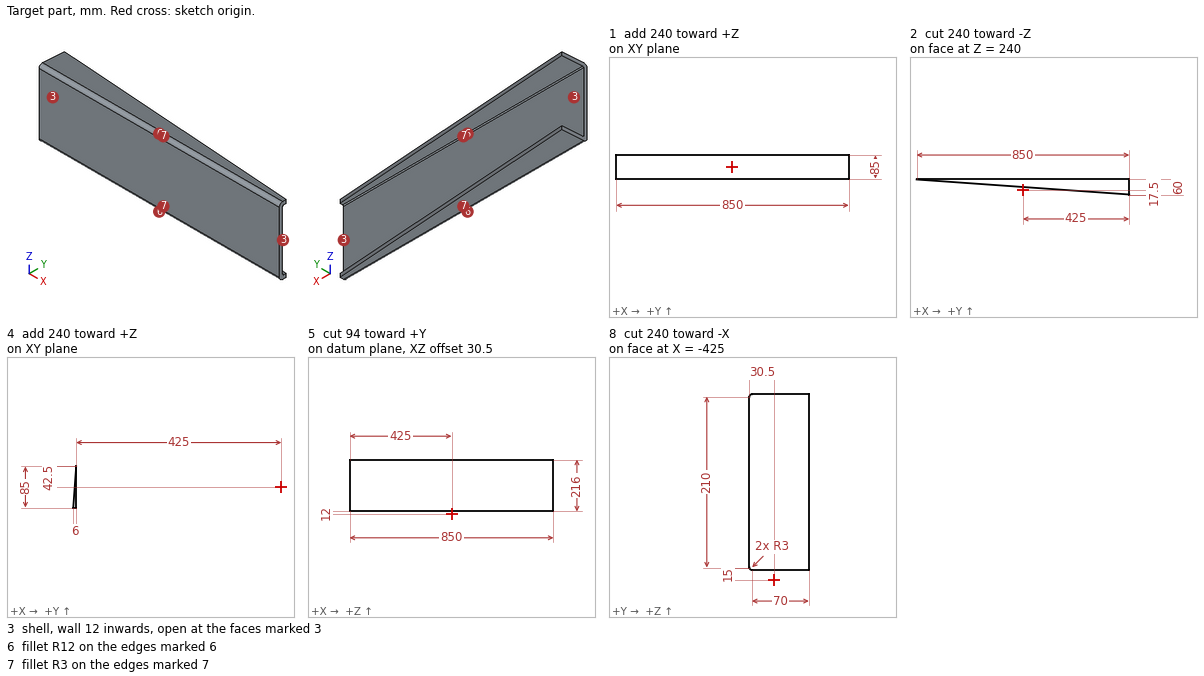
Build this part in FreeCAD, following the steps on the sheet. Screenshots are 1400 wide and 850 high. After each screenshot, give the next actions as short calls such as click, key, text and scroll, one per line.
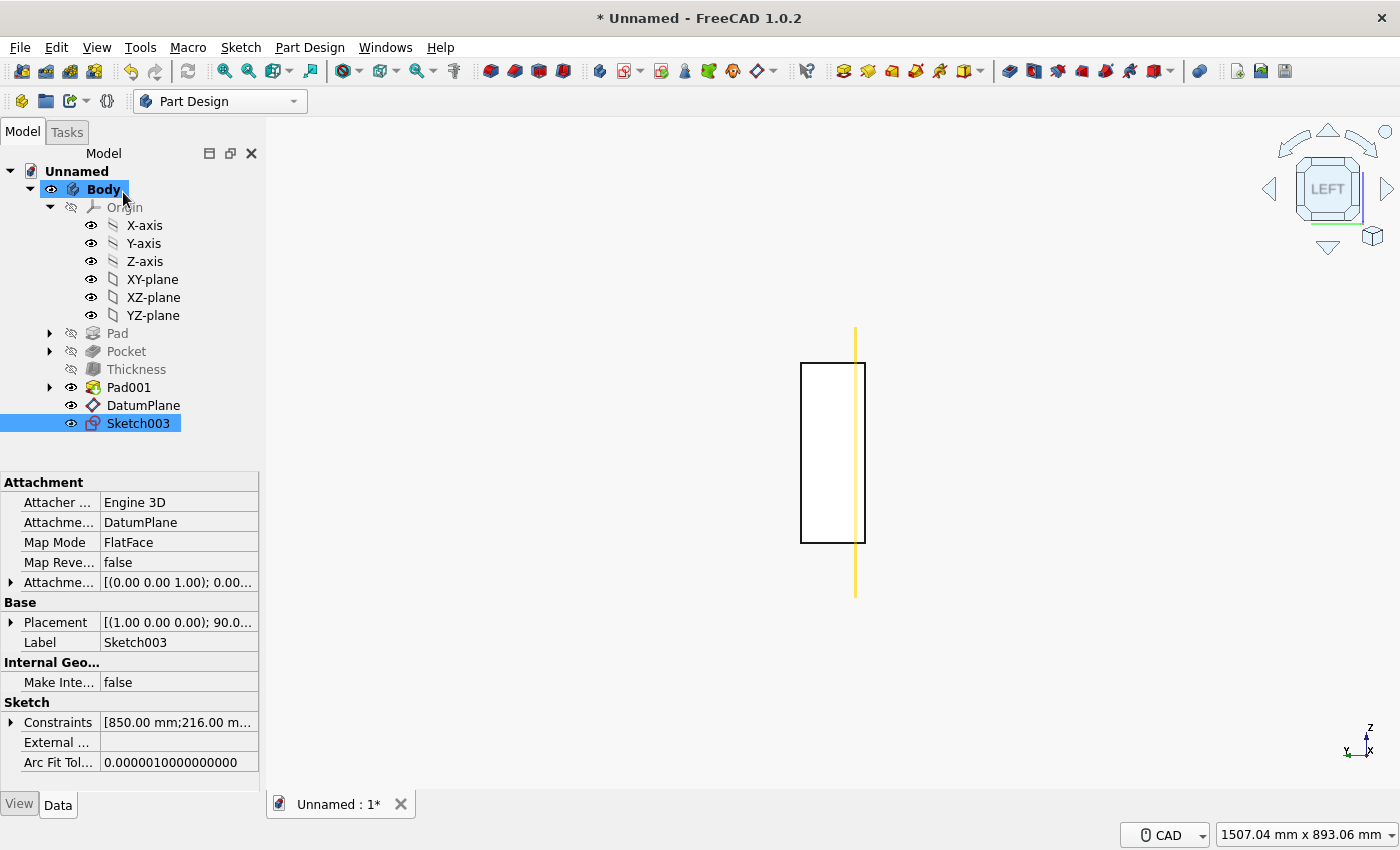
click(1010, 72)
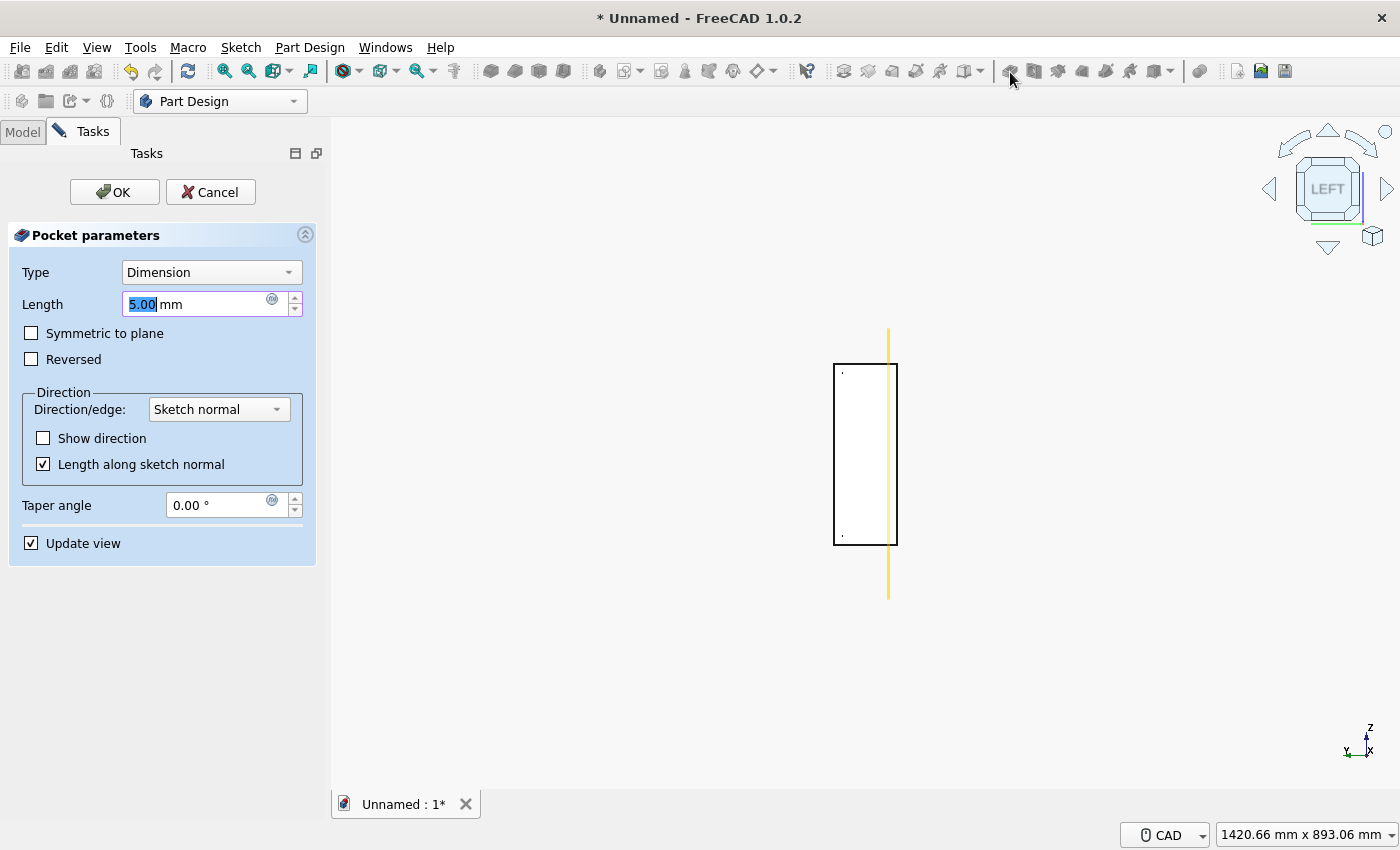
text(94)
key(Tab)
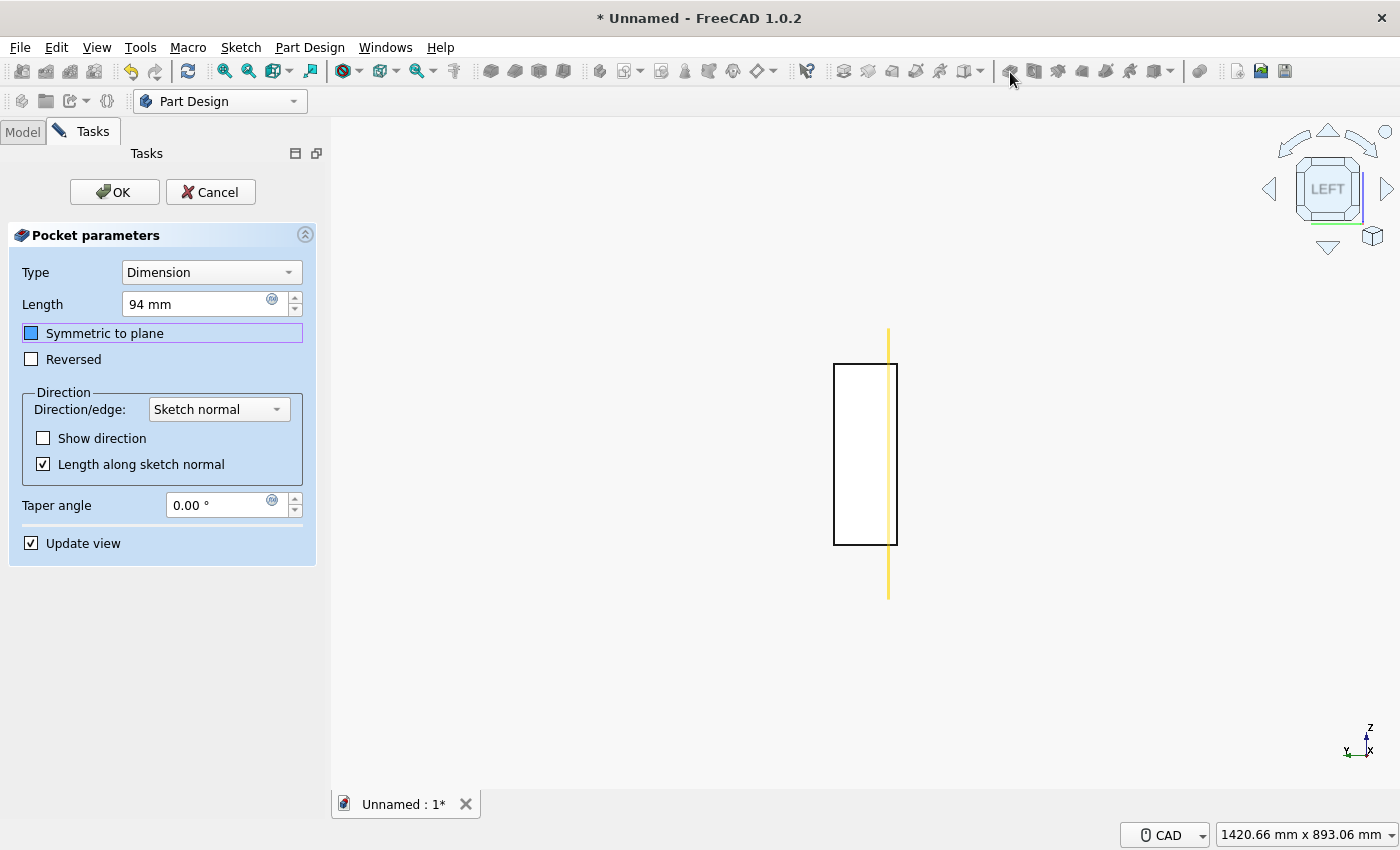
click(115, 192)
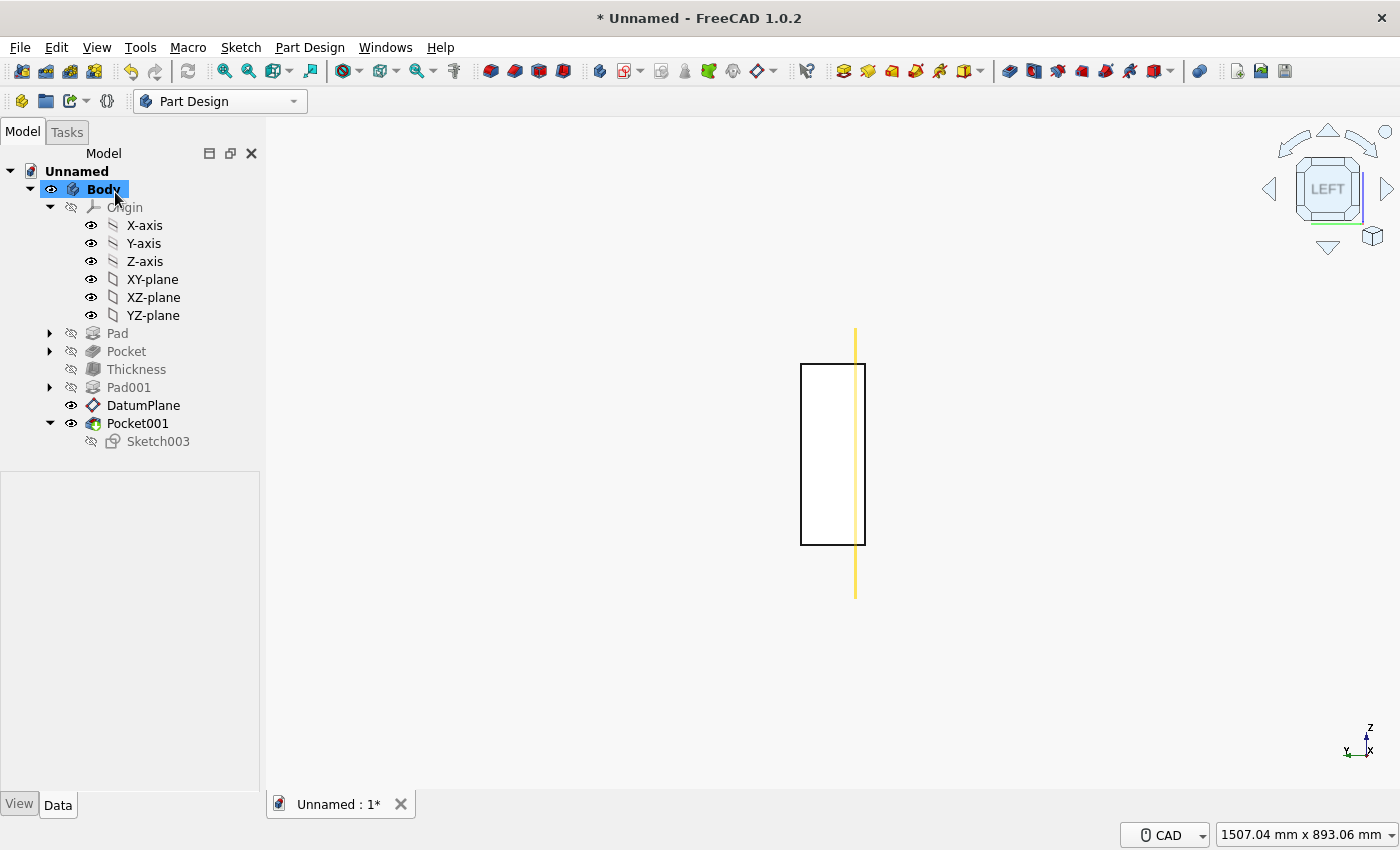
click(116, 405)
key(space)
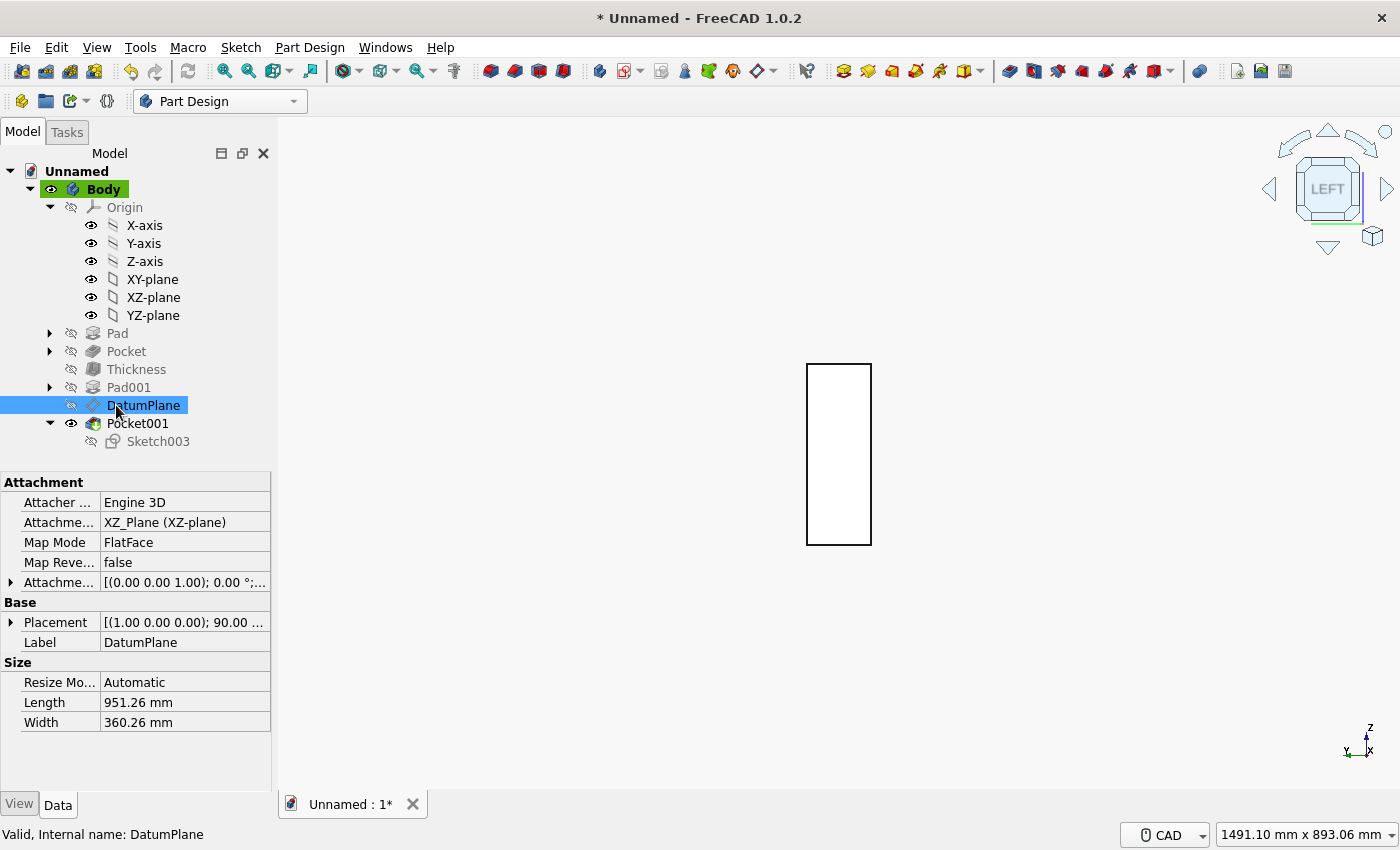
key(v)
key(f)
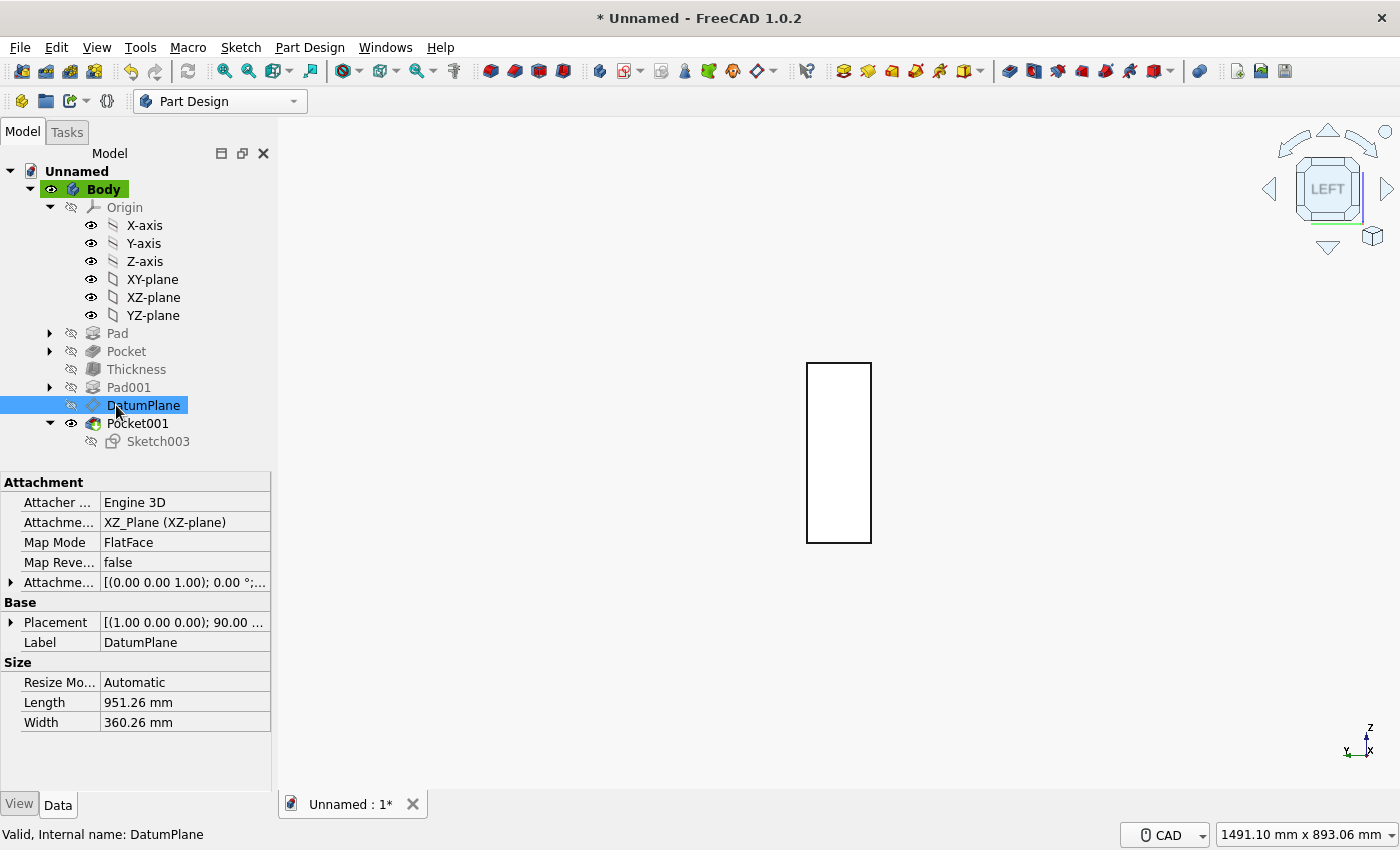
key(0)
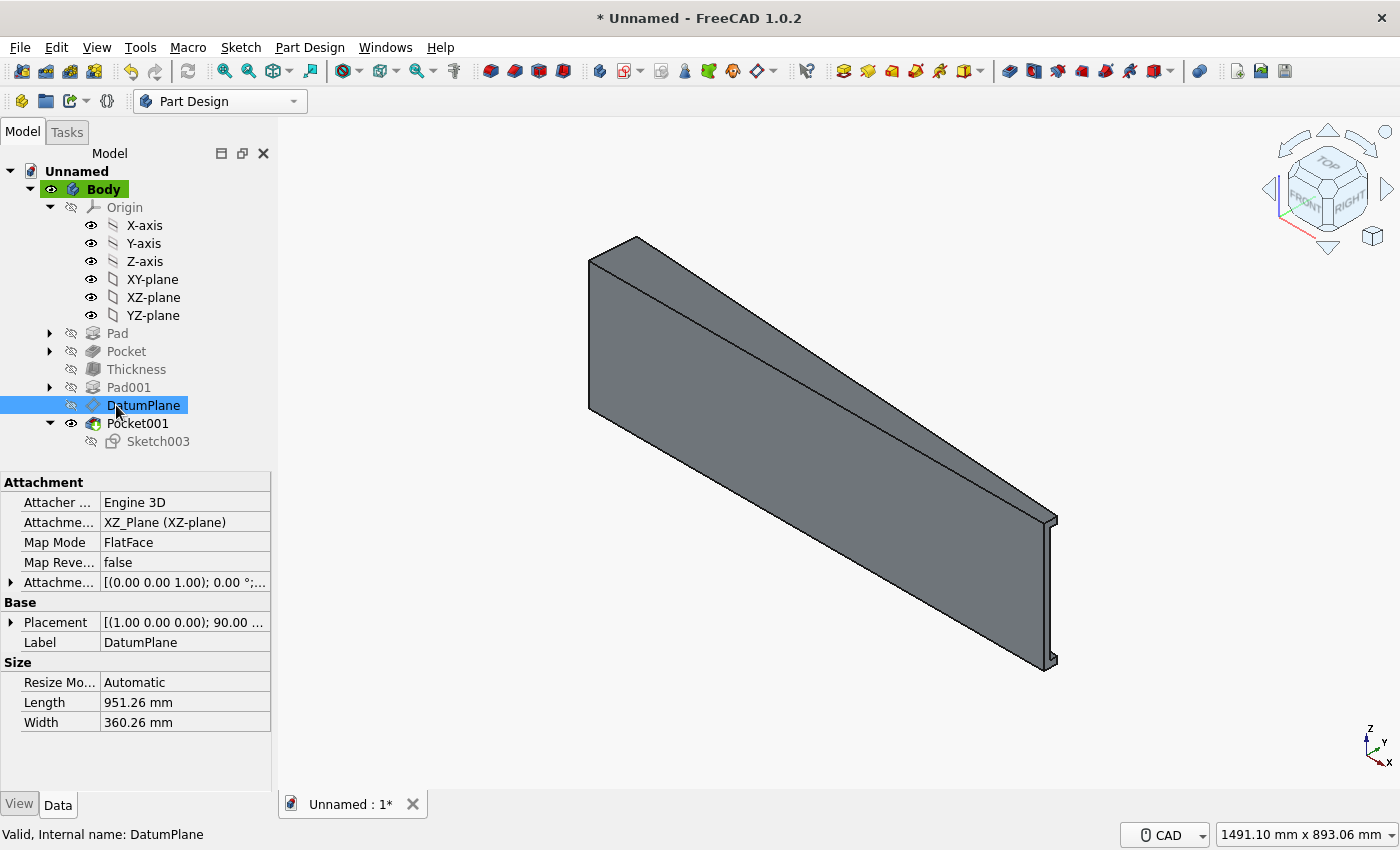
click(816, 391)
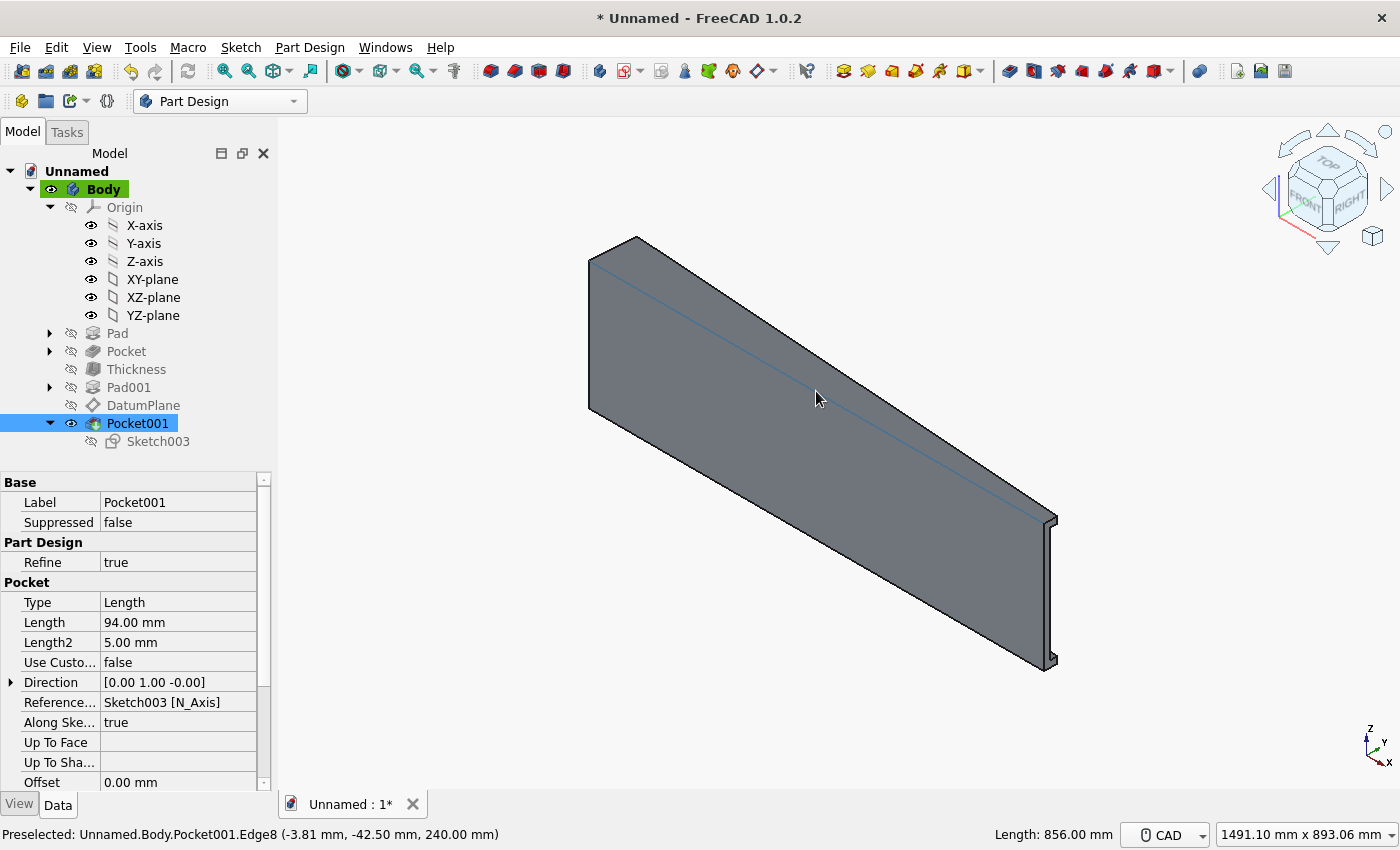
key(2)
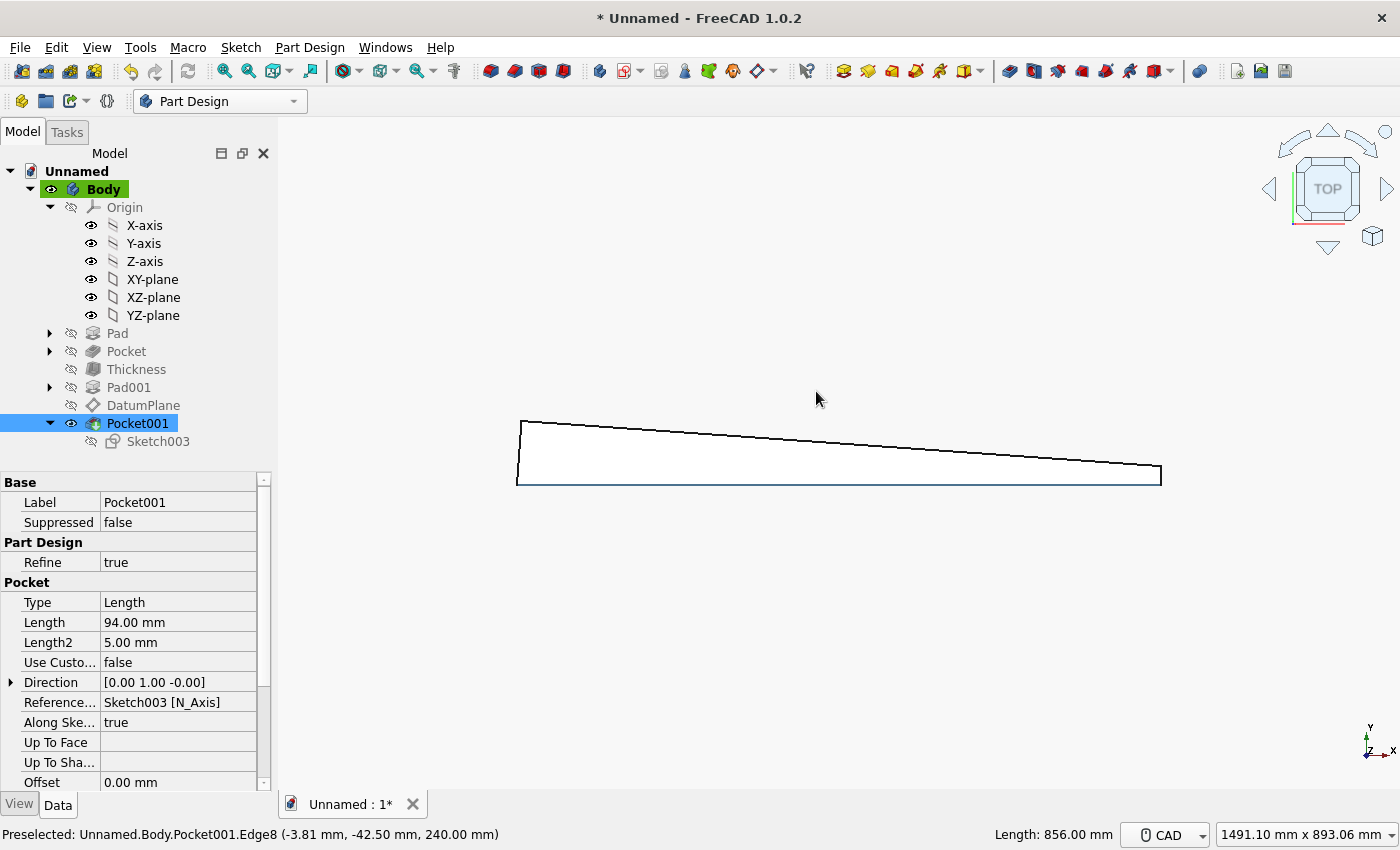
key(1)